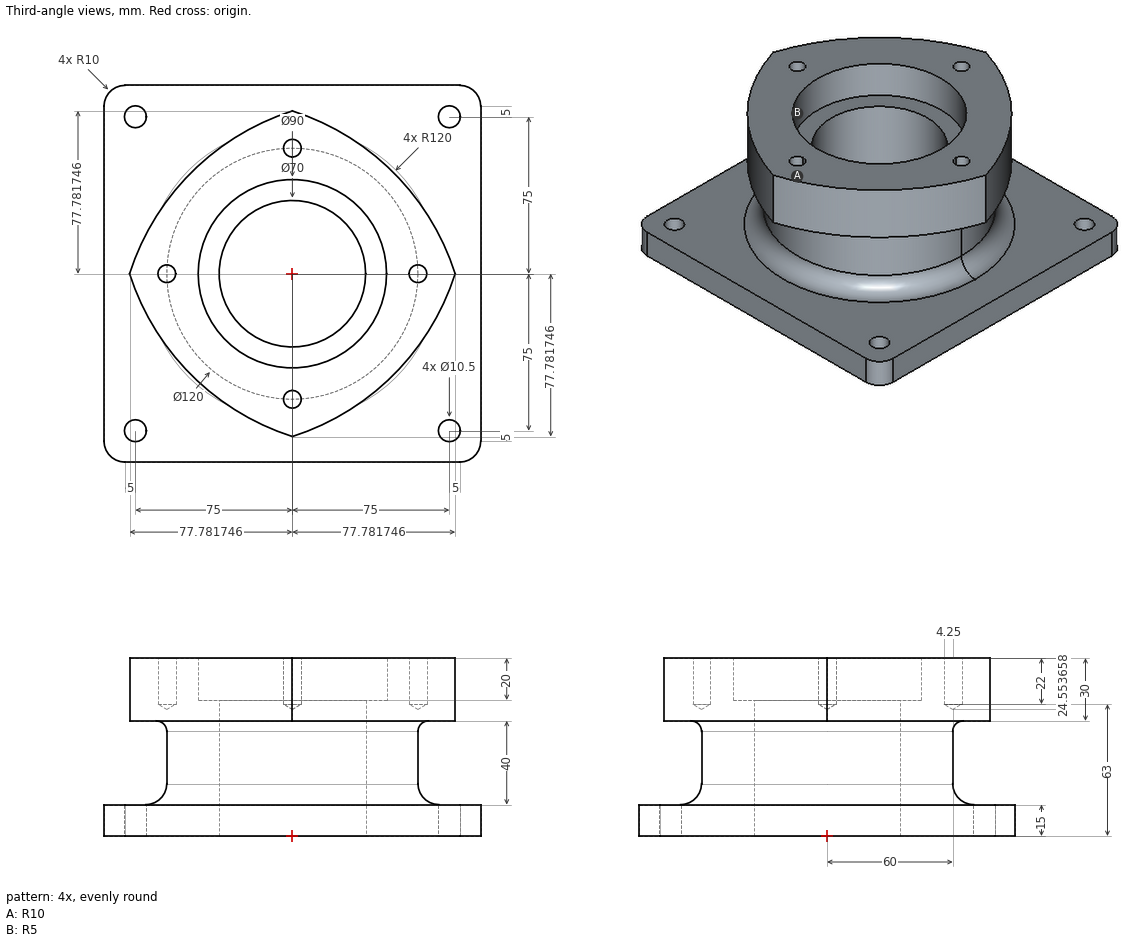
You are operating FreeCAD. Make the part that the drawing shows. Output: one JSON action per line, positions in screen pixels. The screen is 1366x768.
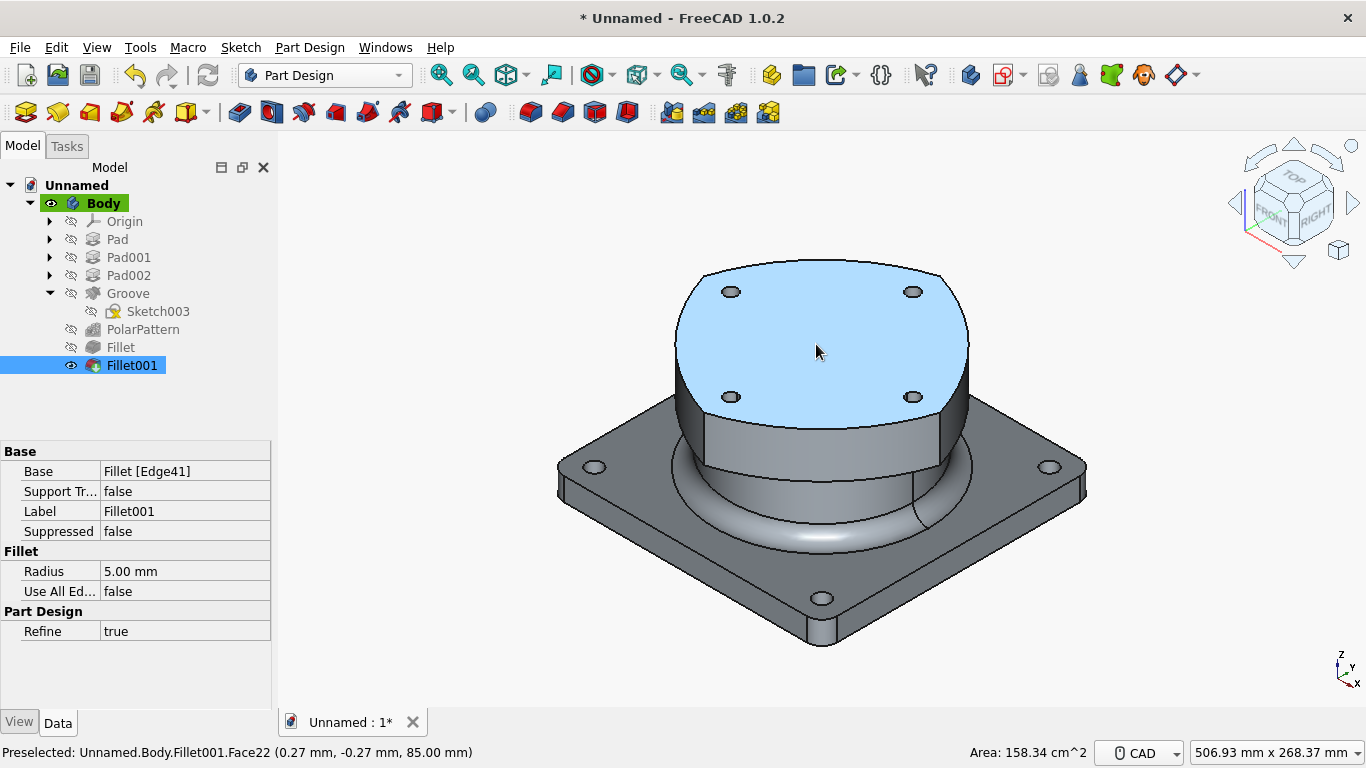
{"action": "left_click", "coordinate": [1004, 76]}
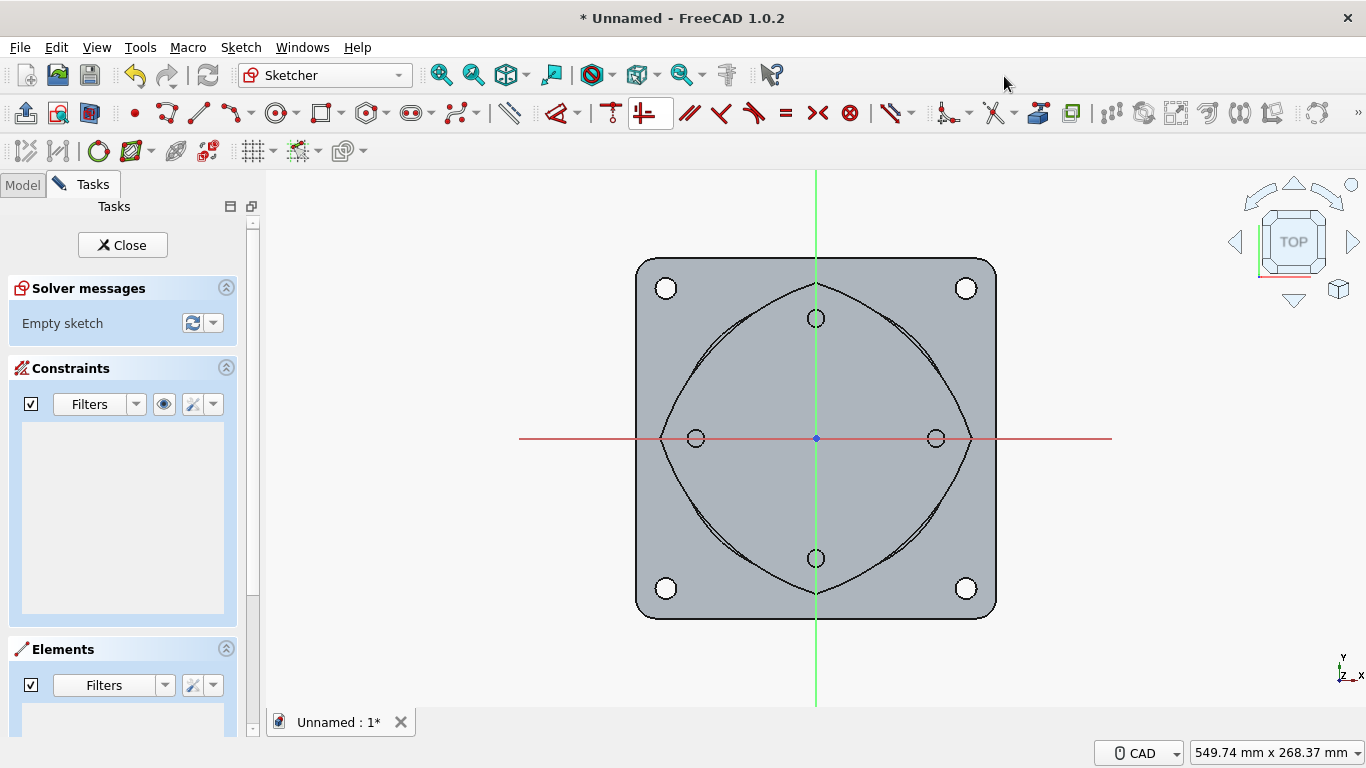
{"action": "scroll", "coordinate": [872, 438], "scroll_direction": "up", "scroll_amount": 4}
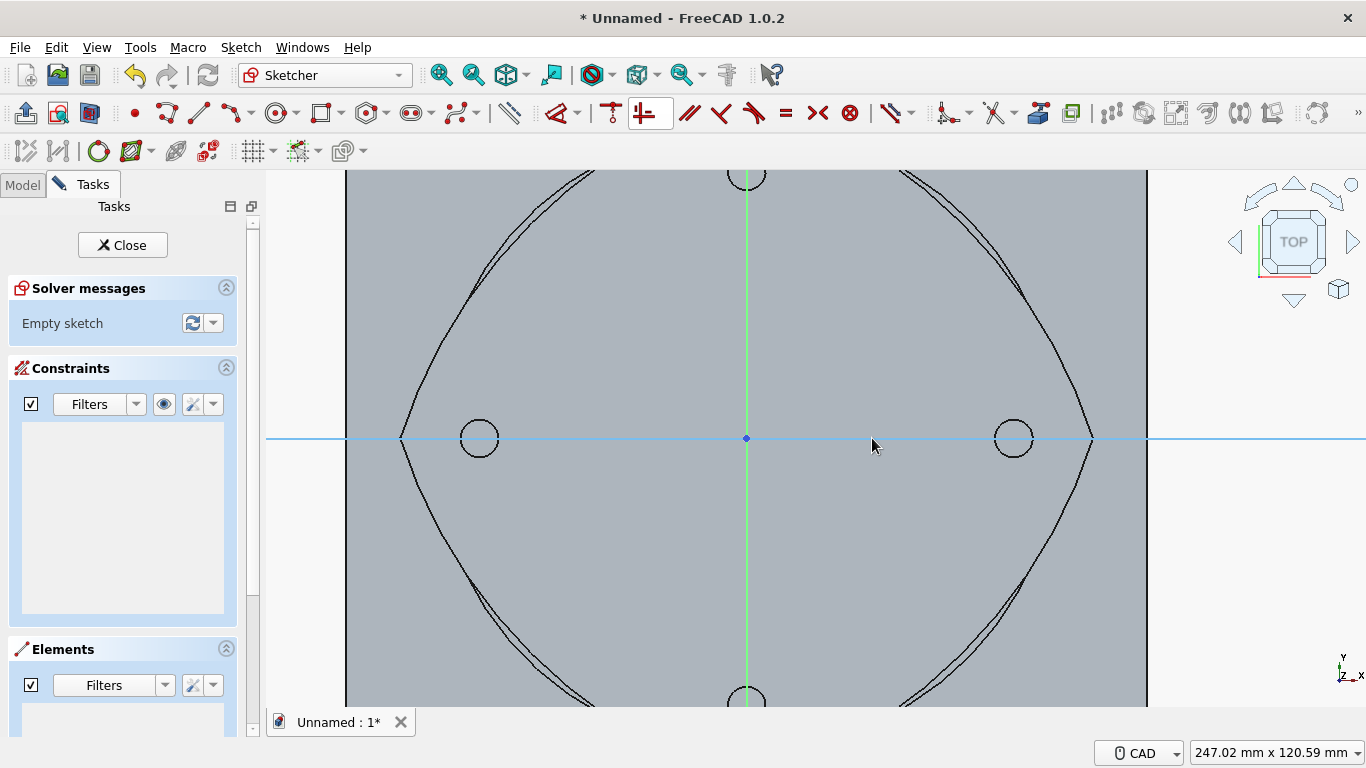
{"action": "left_click", "coordinate": [276, 114]}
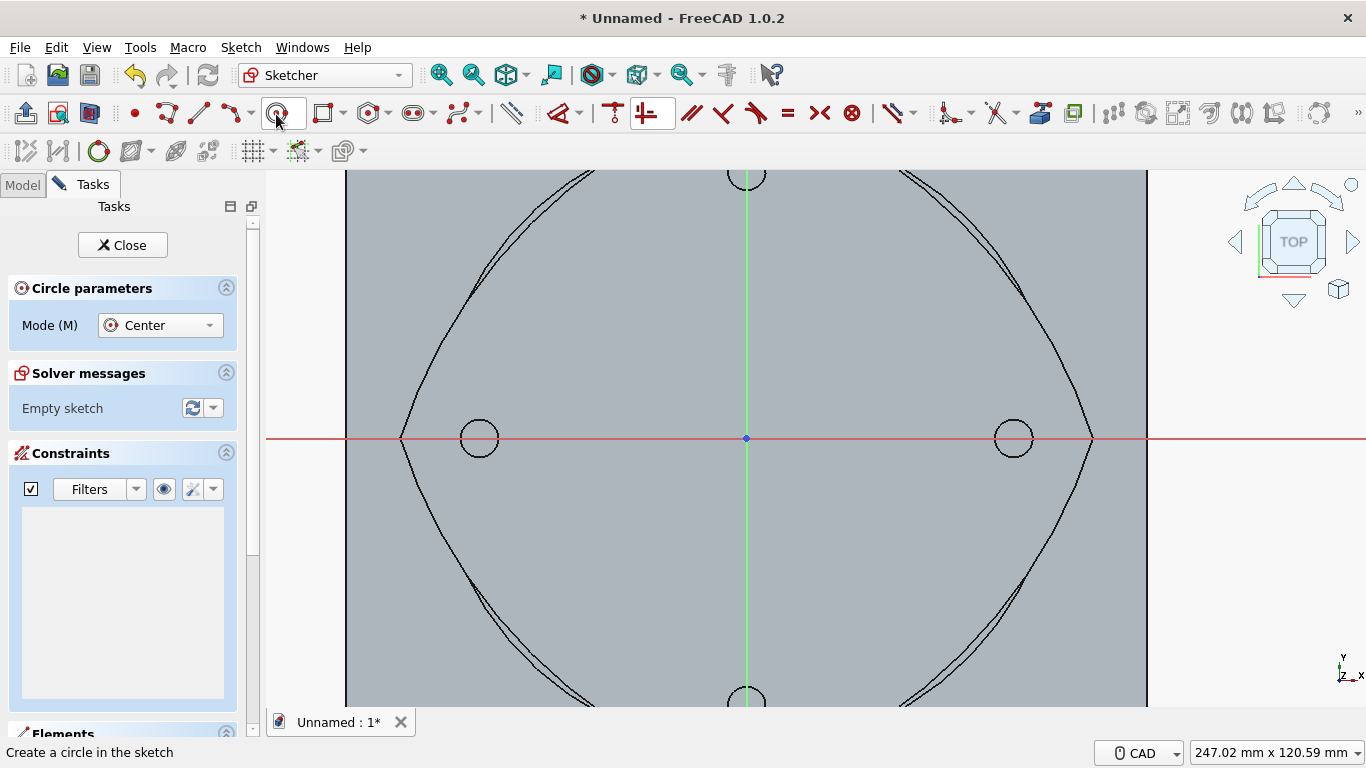
{"action": "left_click", "coordinate": [747, 438]}
{"action": "mouse_move", "coordinate": [857, 328]}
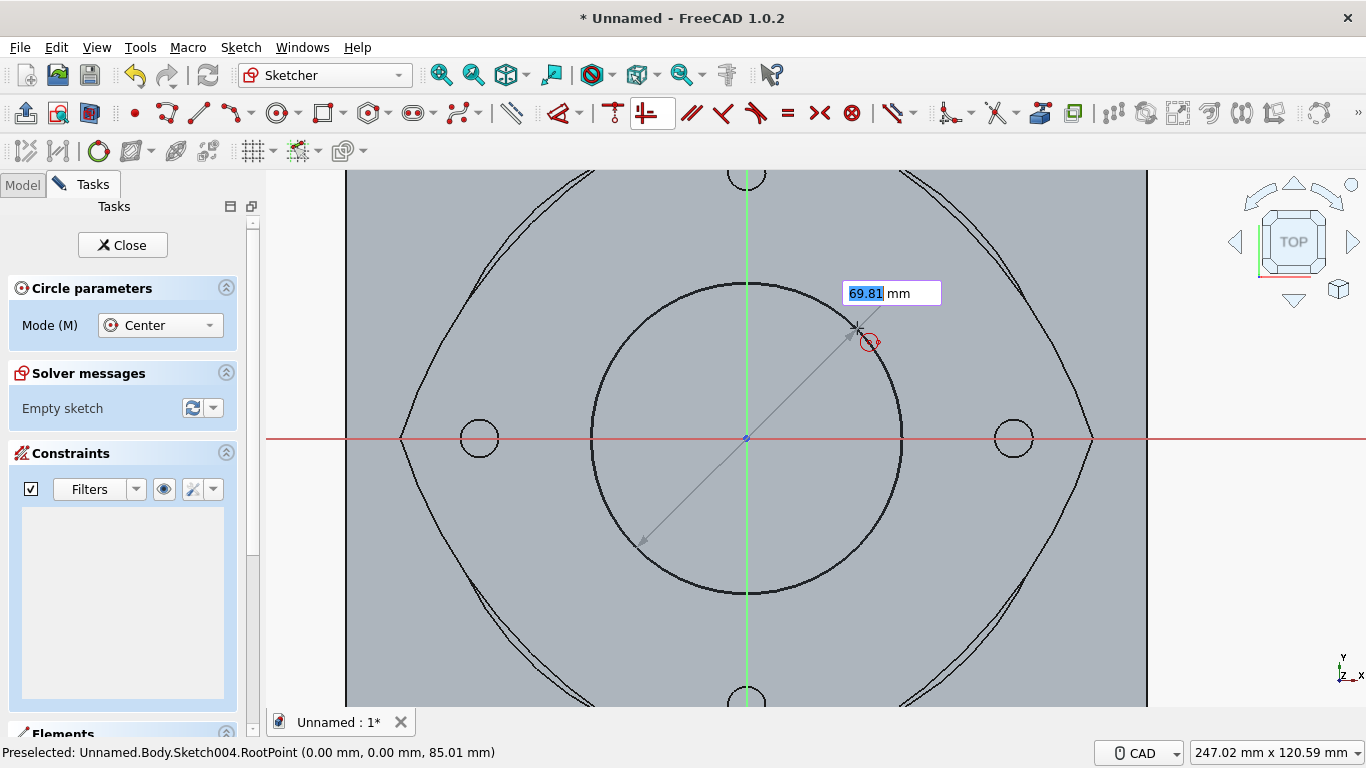
{"action": "type", "text": "70"}
{"action": "key", "text": "Return"}
{"action": "key", "text": "Escape"}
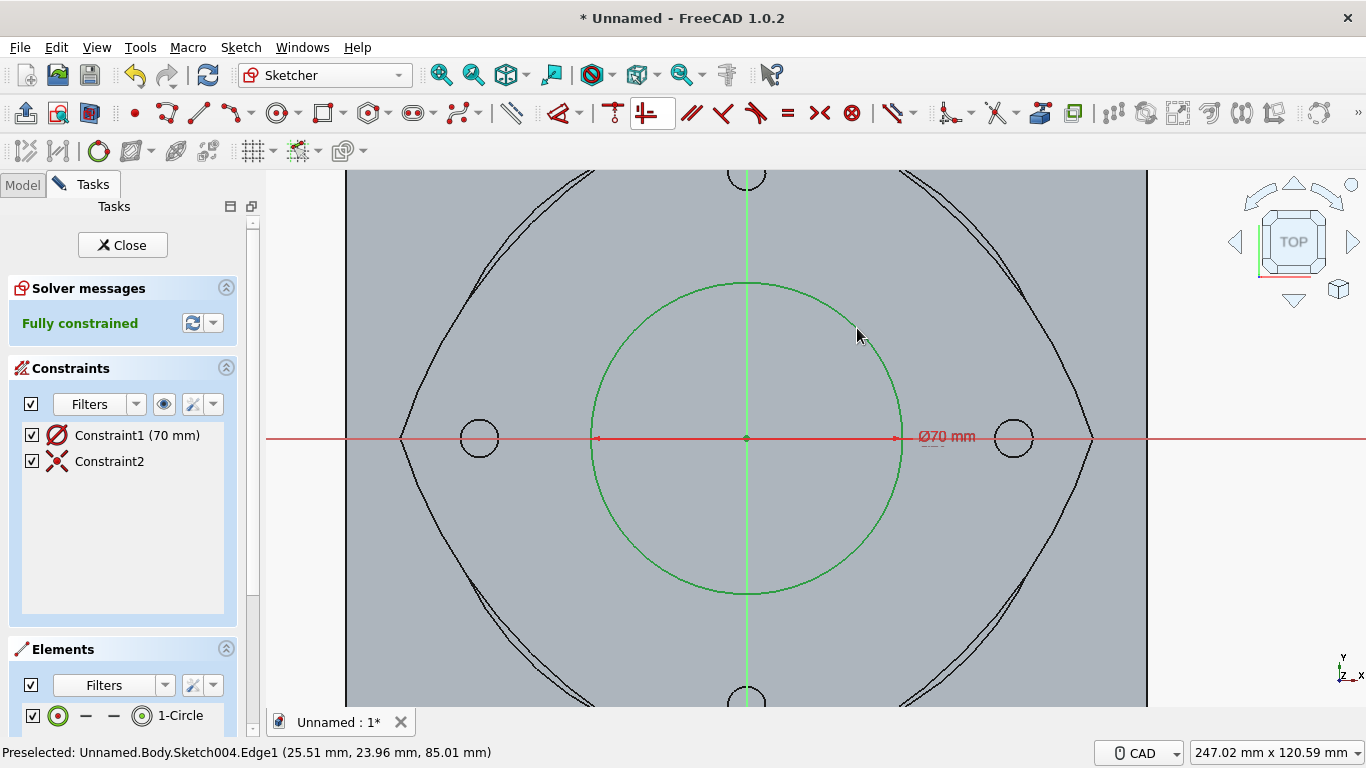
{"action": "left_click", "coordinate": [123, 245]}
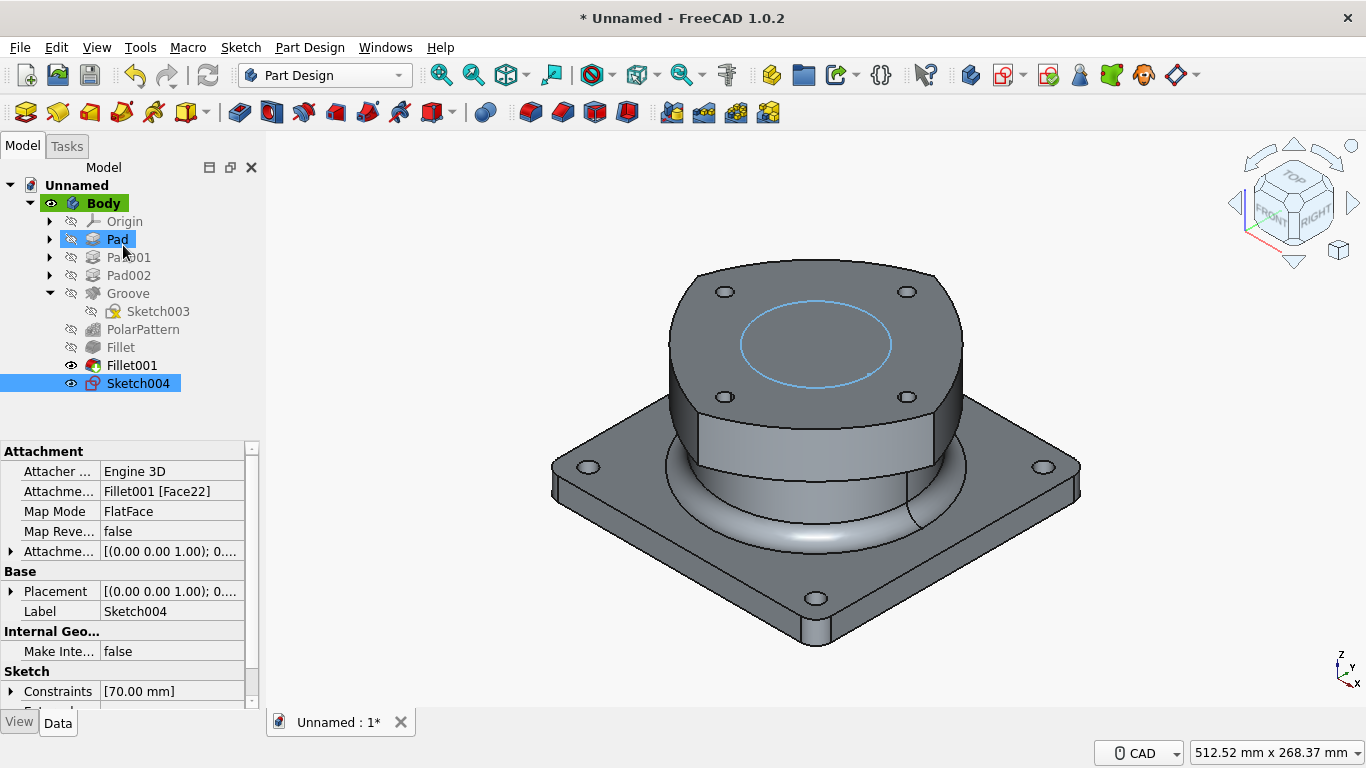
{"action": "left_click", "coordinate": [240, 112]}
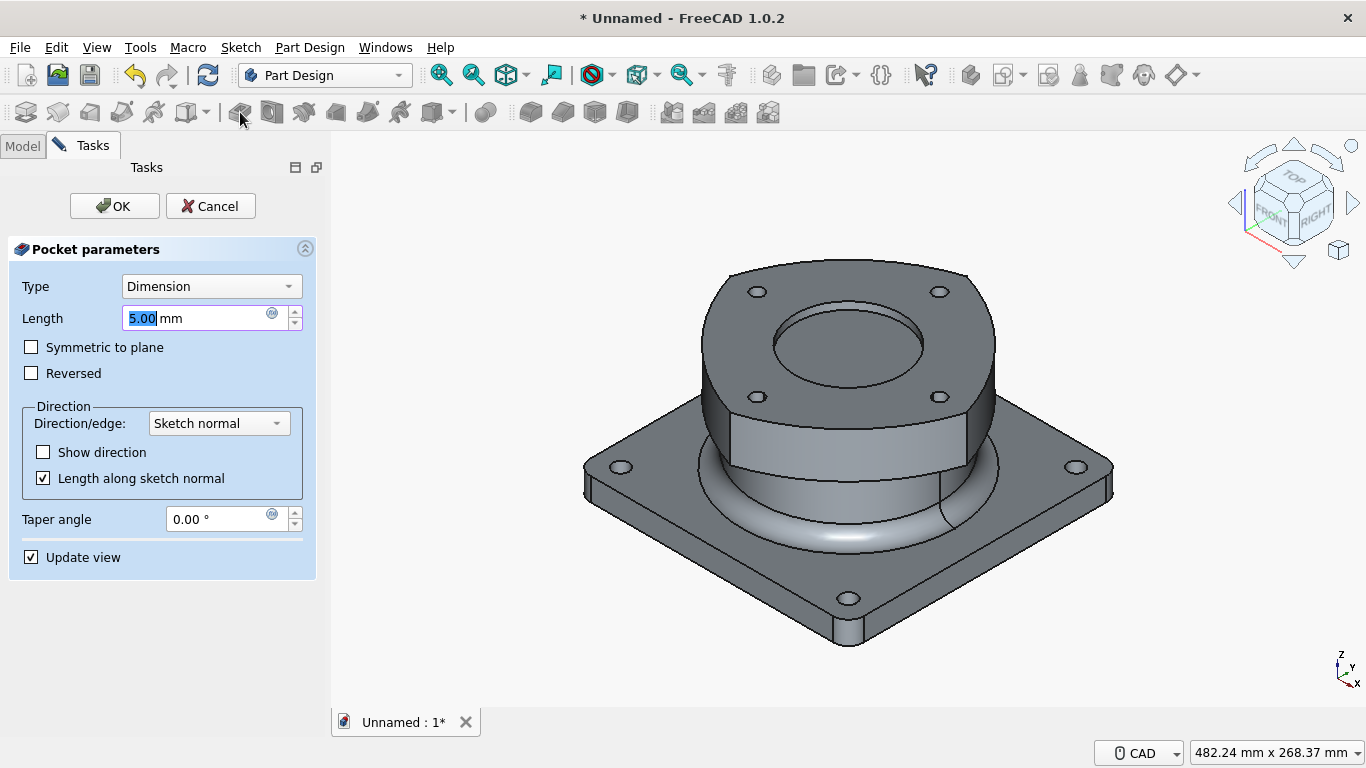
{"action": "left_click", "coordinate": [212, 286]}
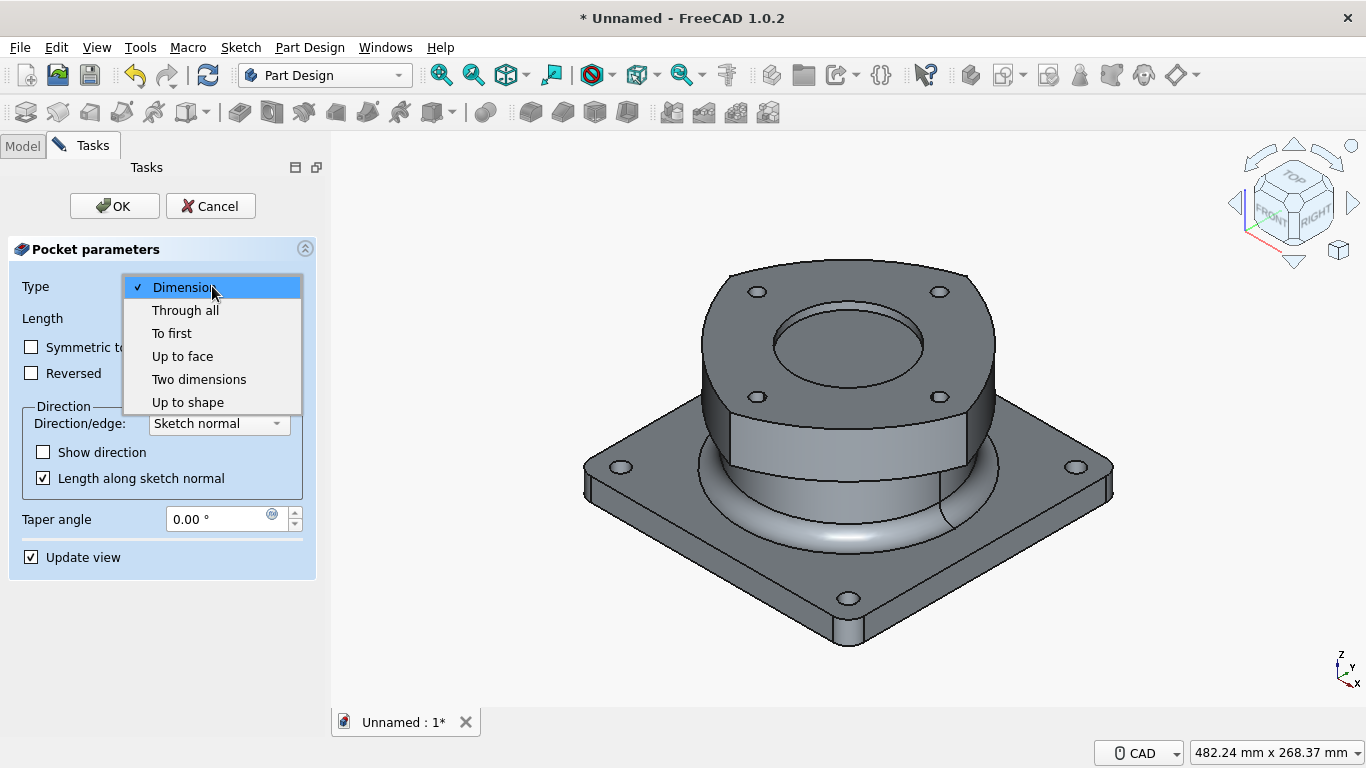
{"action": "left_click", "coordinate": [212, 310]}